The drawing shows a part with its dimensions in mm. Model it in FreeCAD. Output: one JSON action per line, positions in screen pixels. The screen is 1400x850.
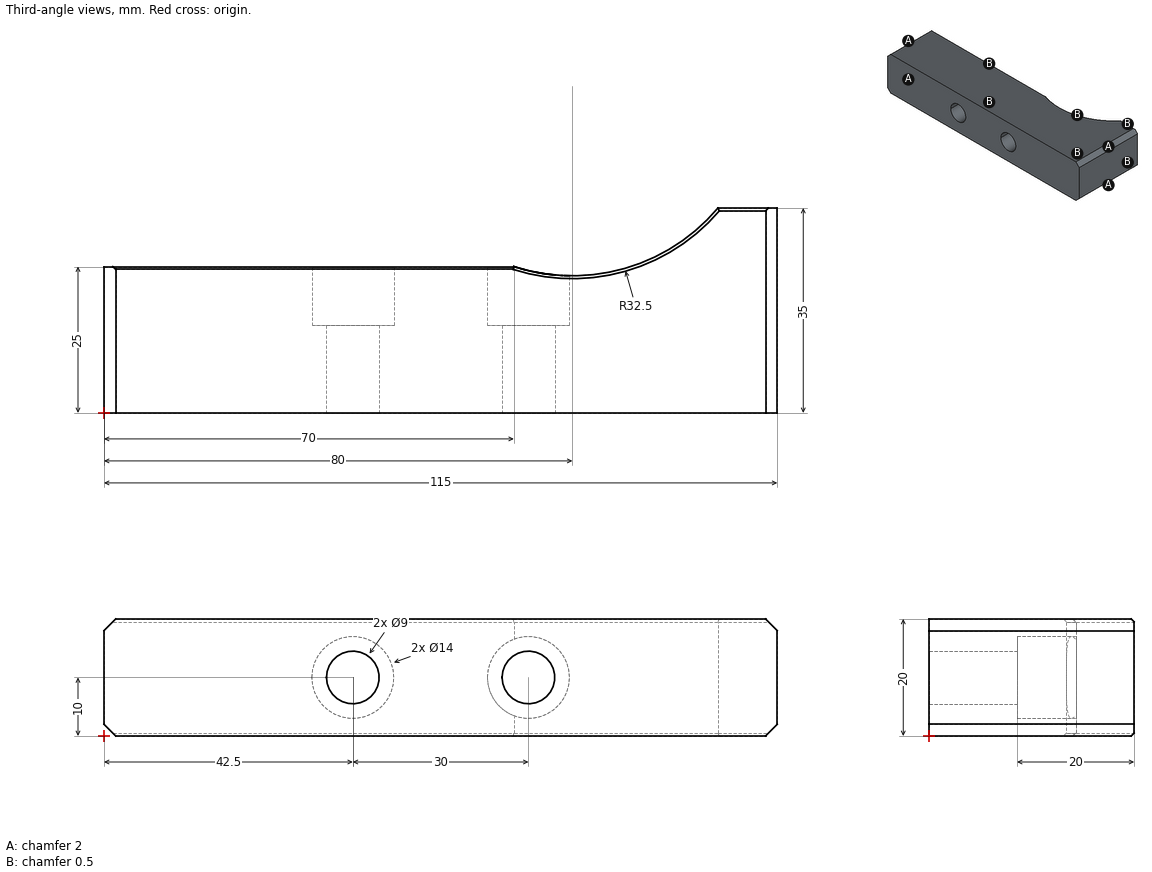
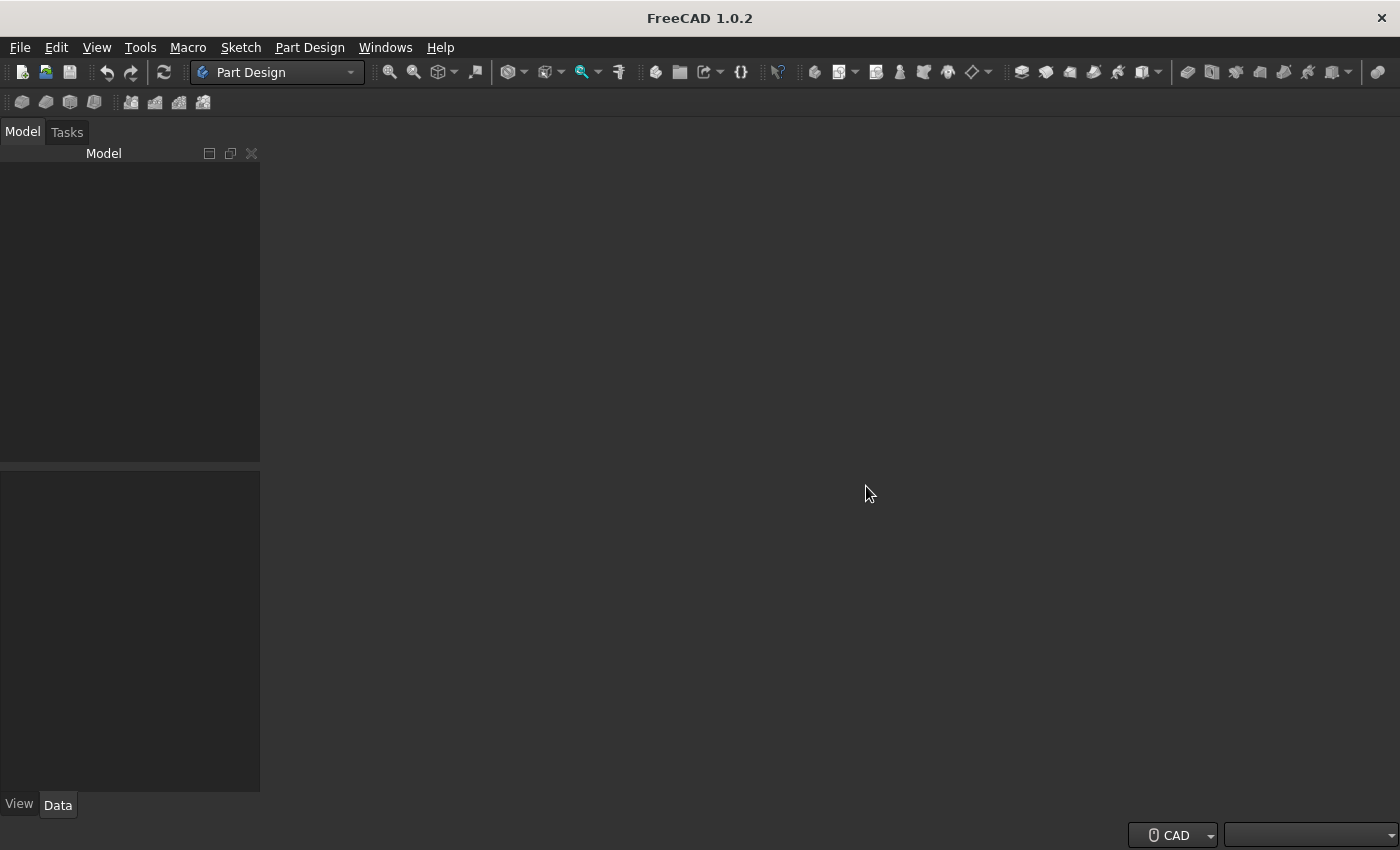
{"action": "left_click", "coordinate": [22, 72]}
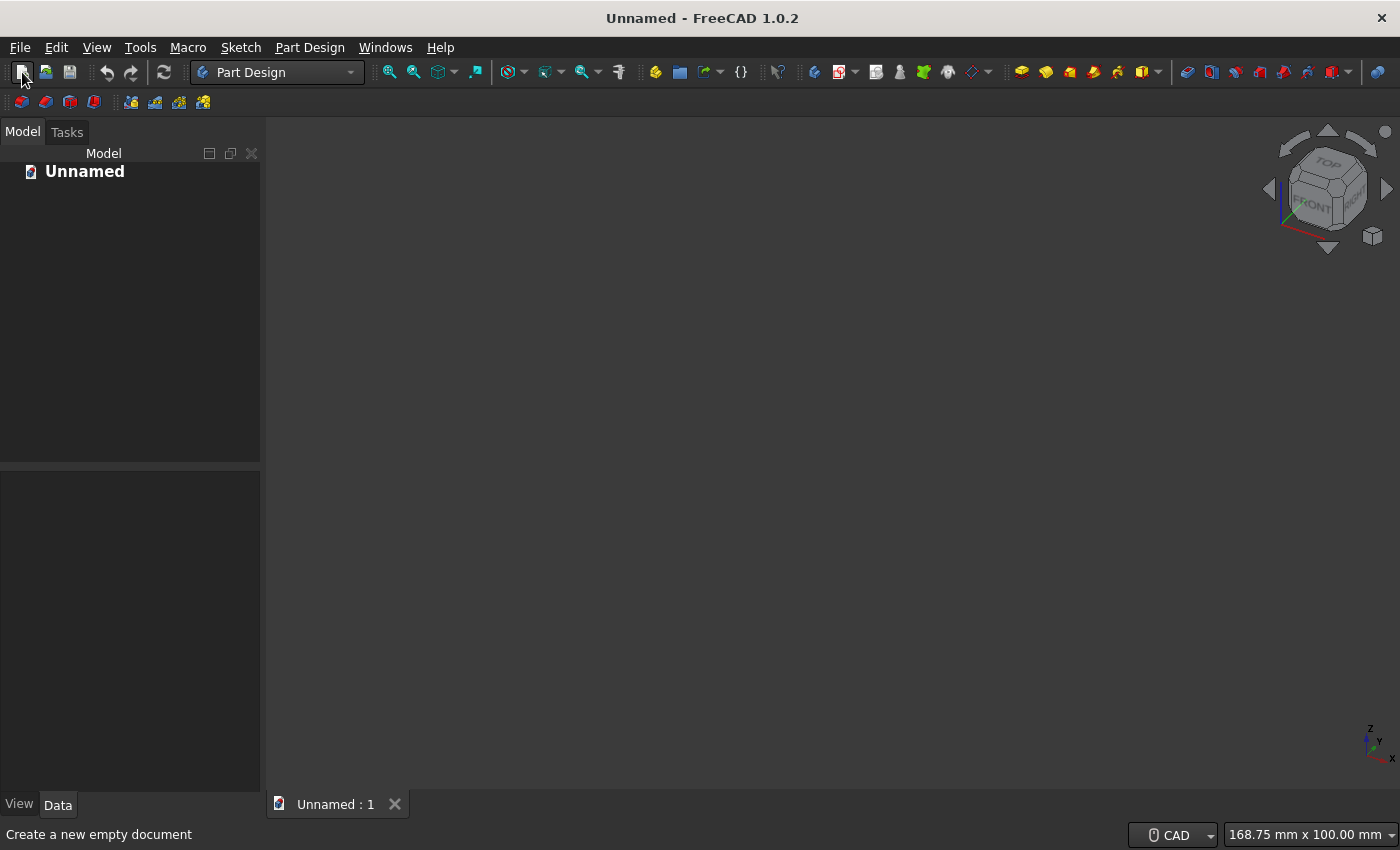
{"action": "left_click", "coordinate": [840, 72]}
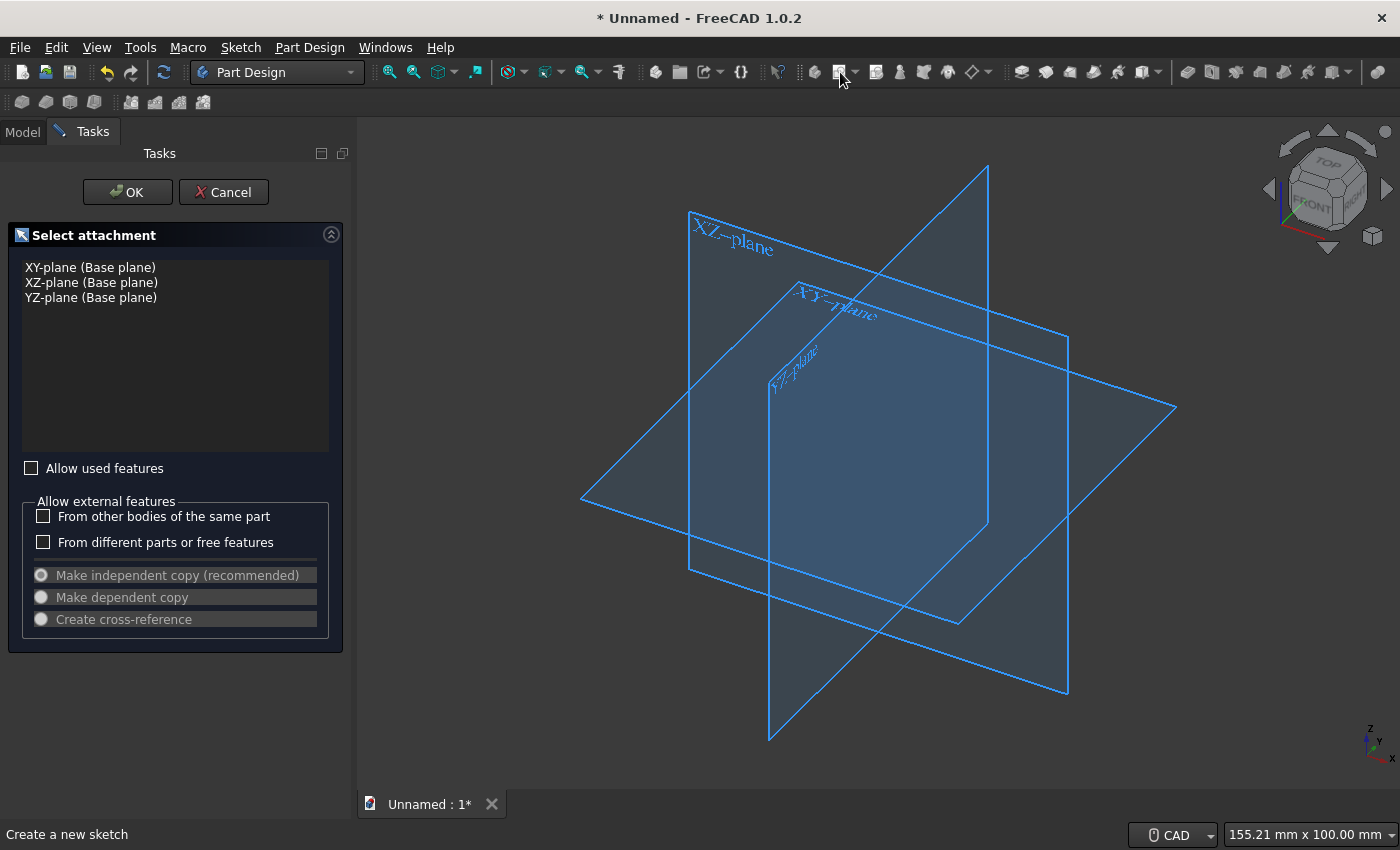
{"action": "left_click", "coordinate": [82, 268]}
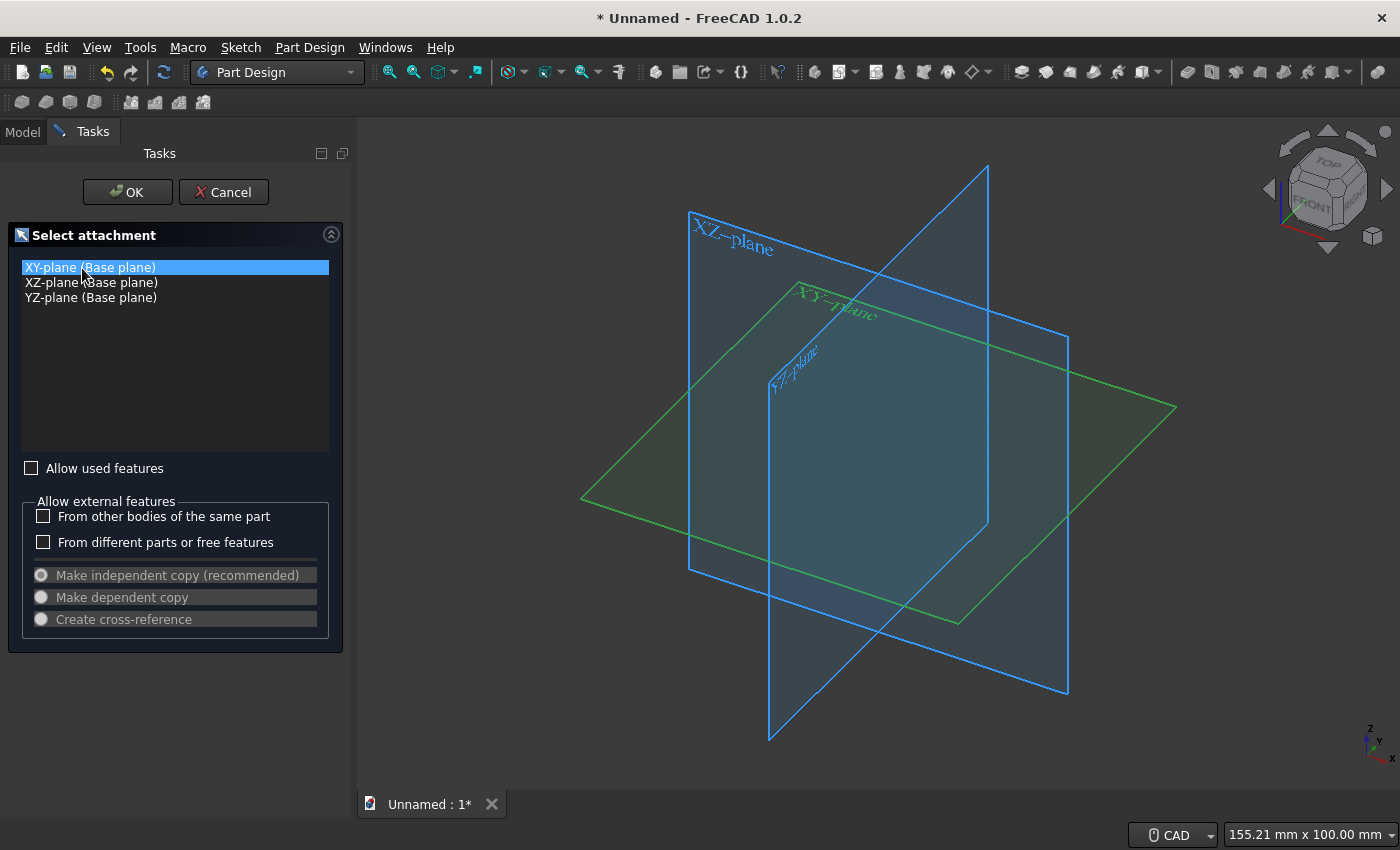
{"action": "left_click", "coordinate": [128, 192]}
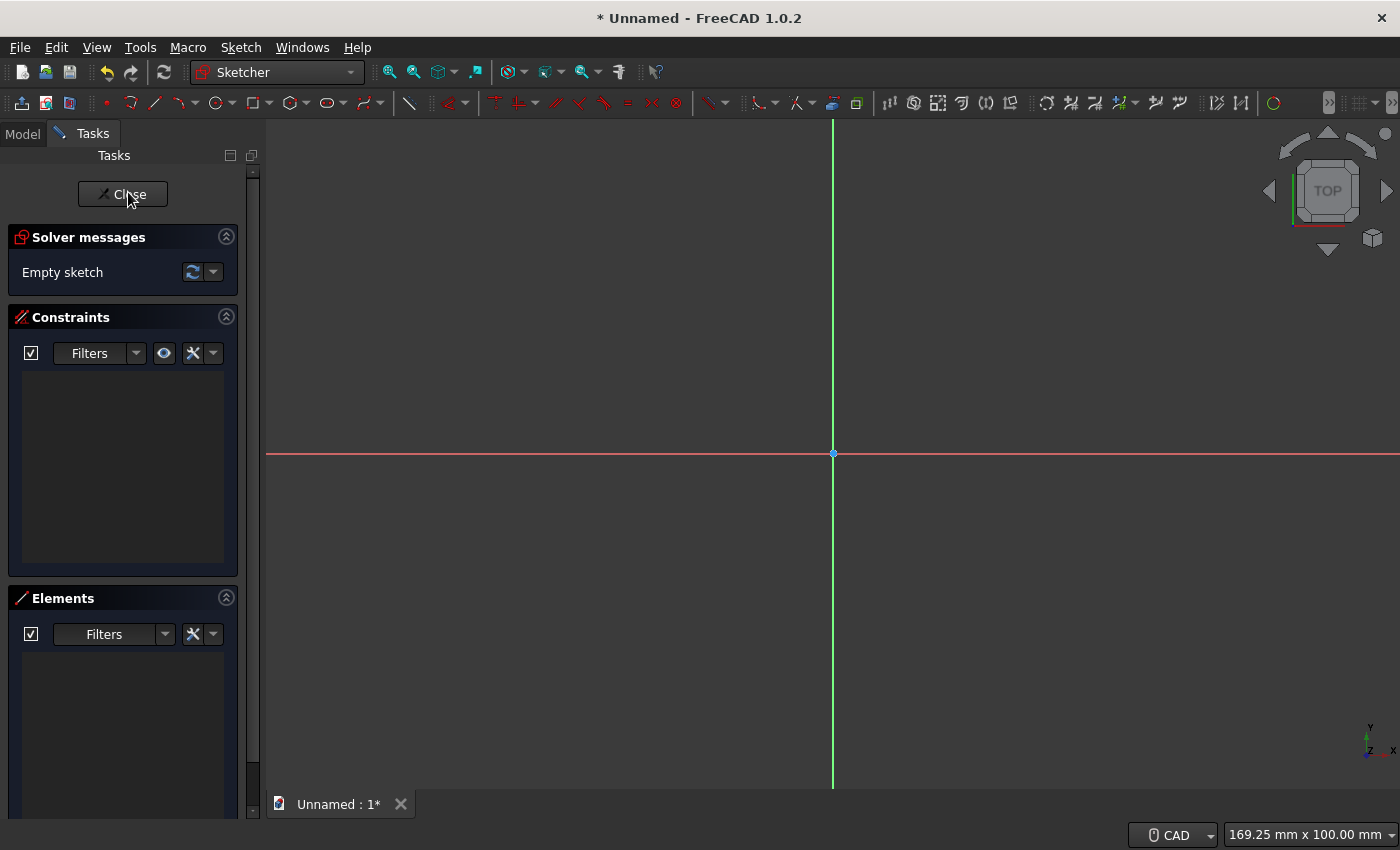
{"action": "scroll", "coordinate": [294, 692], "scroll_direction": "down", "scroll_amount": 2}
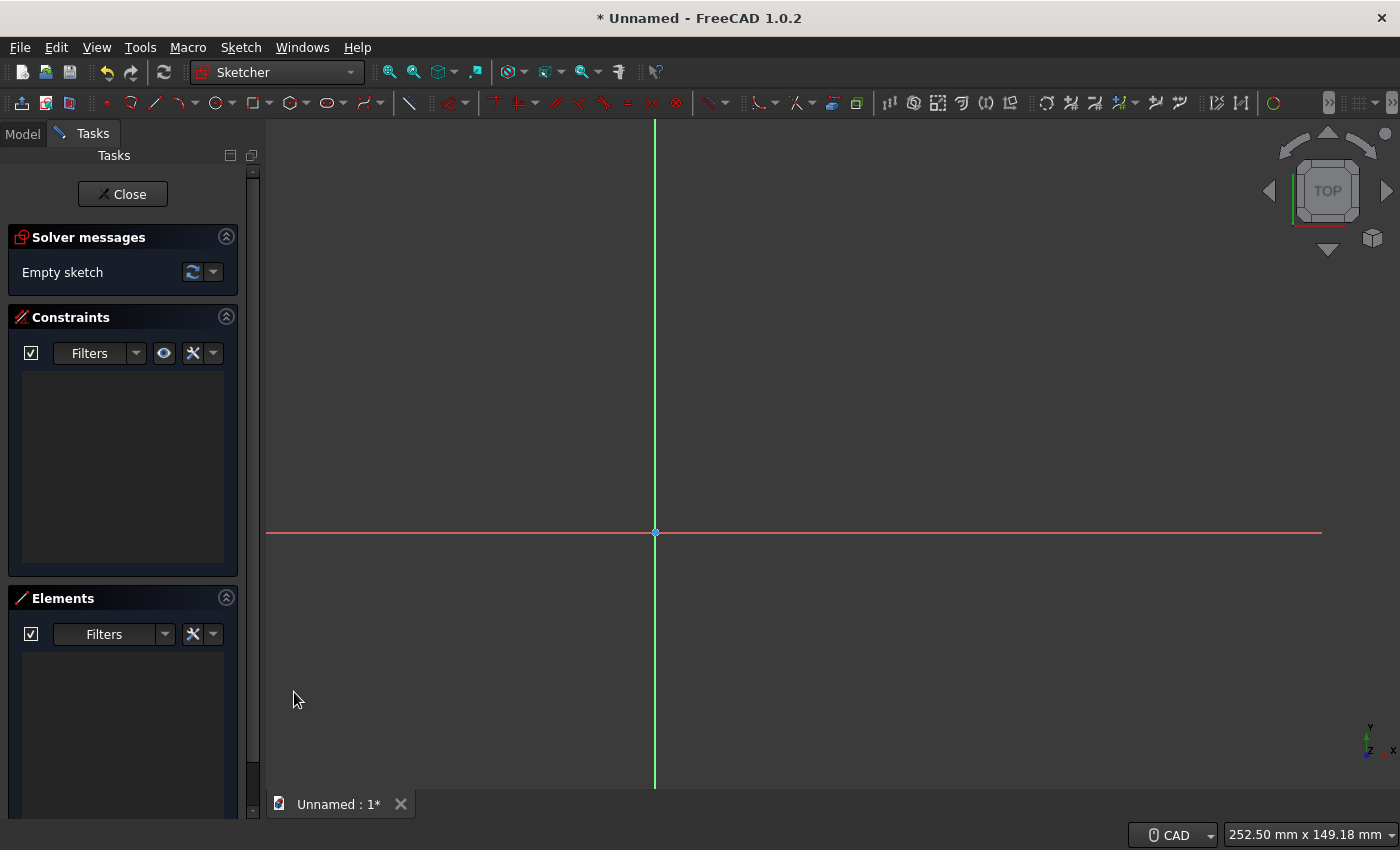
{"action": "left_click", "coordinate": [132, 104]}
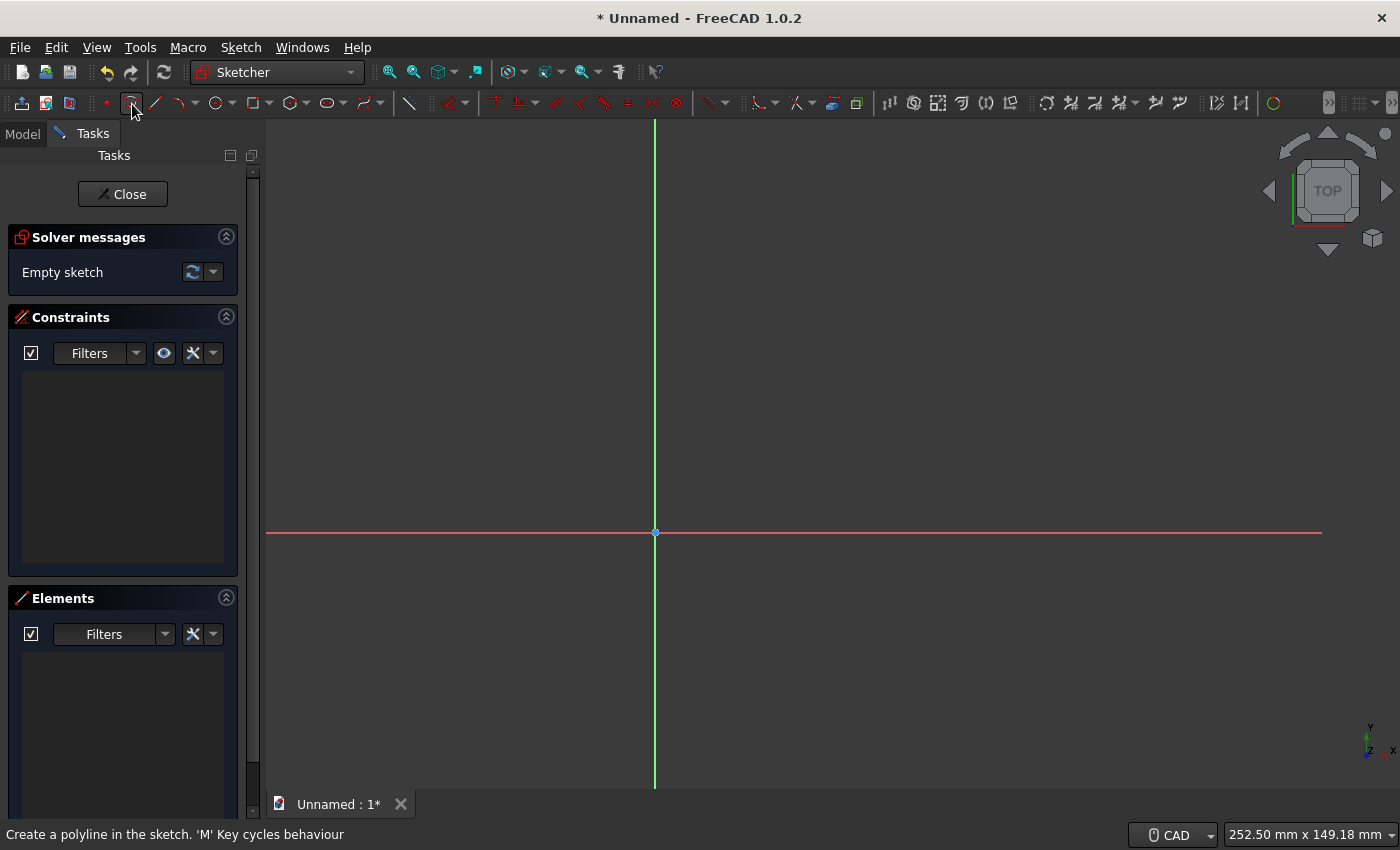
{"action": "left_click", "coordinate": [970, 420]}
{"action": "left_click", "coordinate": [655, 420]}
{"action": "left_click", "coordinate": [655, 533]}
{"action": "left_click", "coordinate": [1172, 524]}
{"action": "left_click", "coordinate": [1172, 376]}
{"action": "left_click", "coordinate": [1126, 376]}
{"action": "right_click", "coordinate": [1126, 376]}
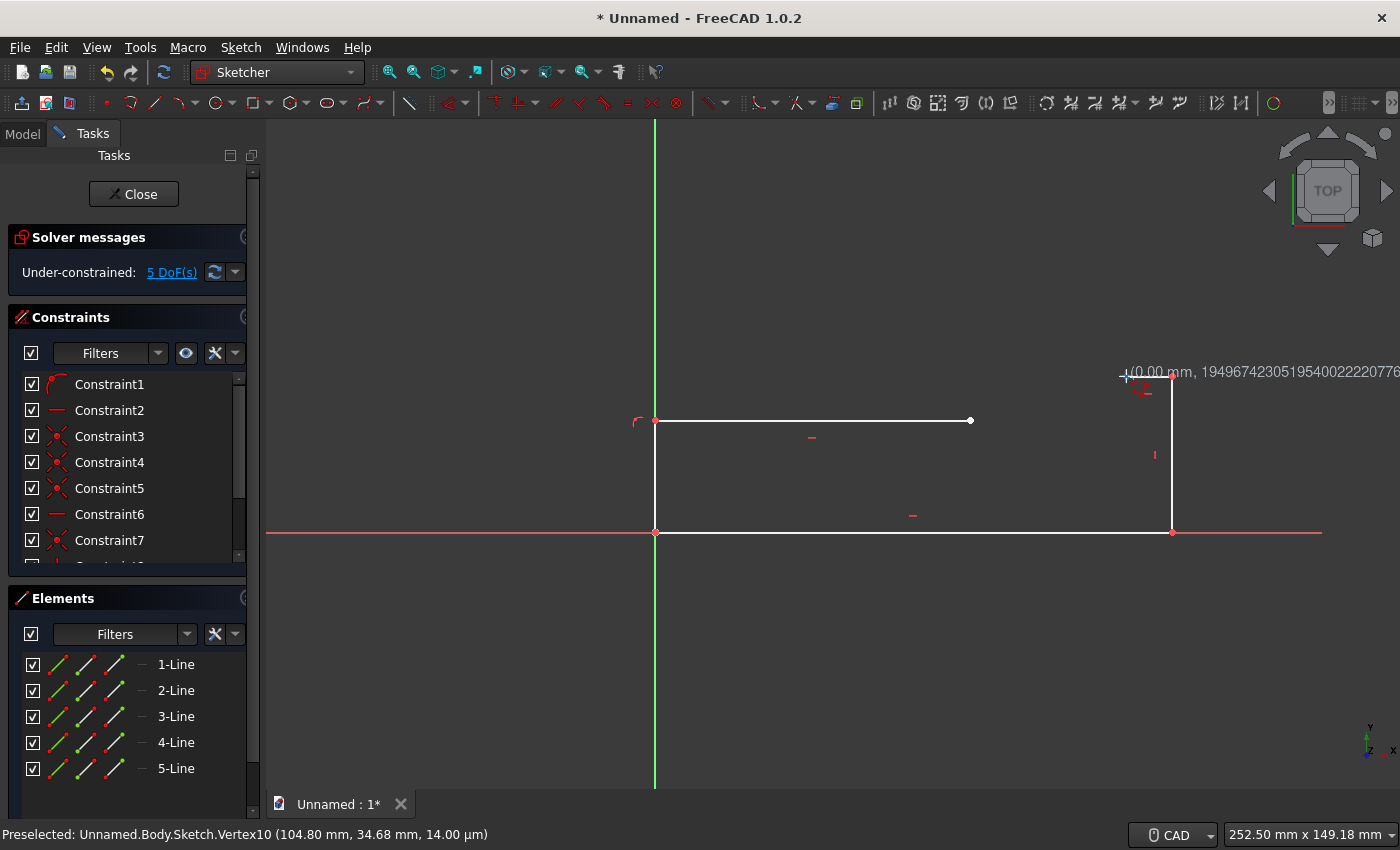
{"action": "left_click", "coordinate": [180, 104]}